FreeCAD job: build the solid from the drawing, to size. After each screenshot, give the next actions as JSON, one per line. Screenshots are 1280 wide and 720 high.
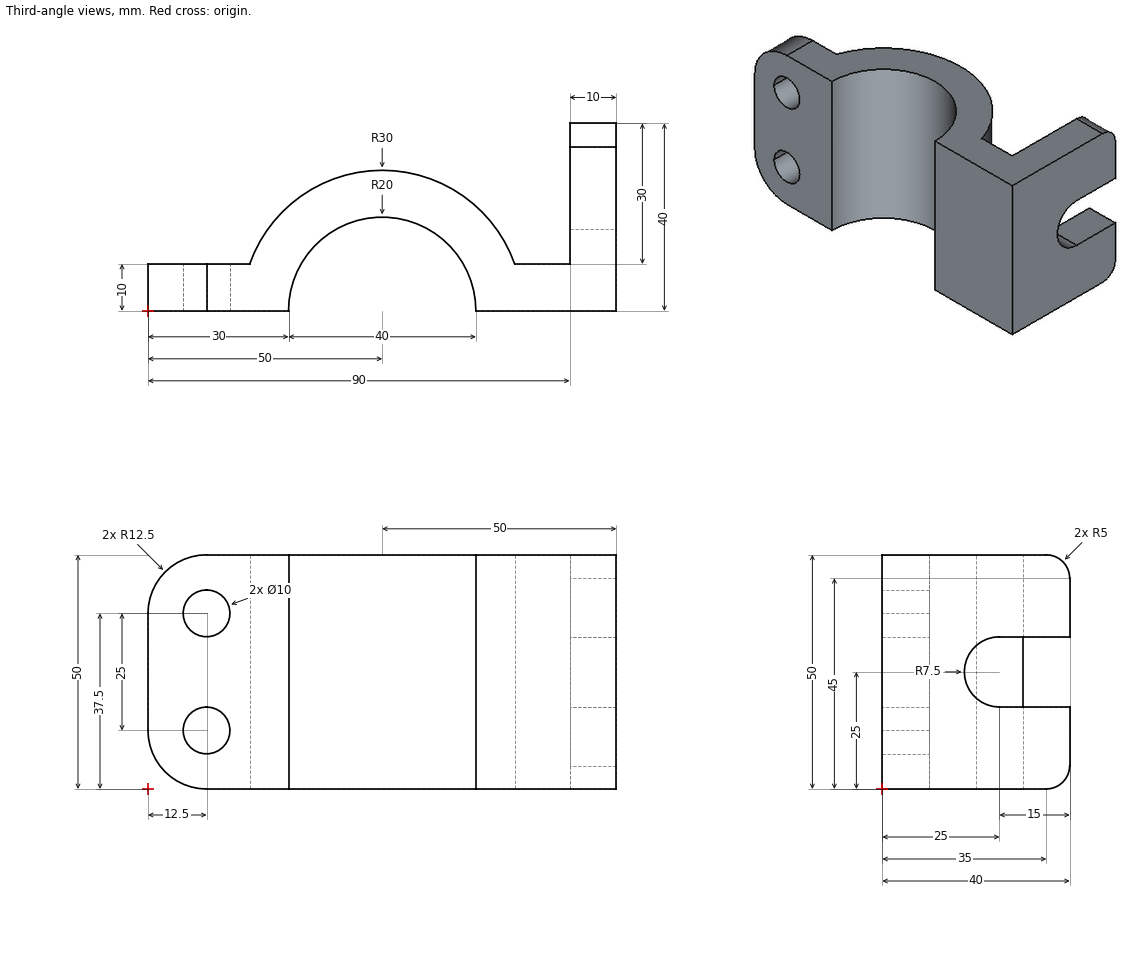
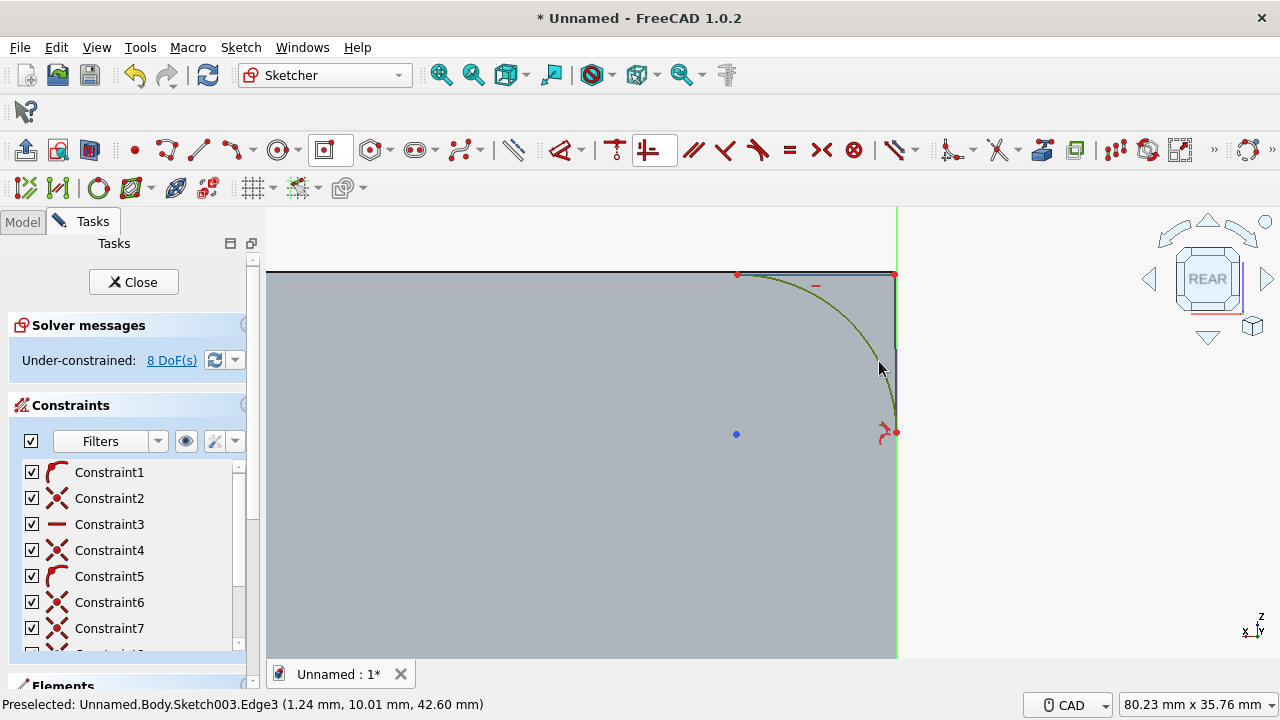
{"action": "left_click", "coordinate": [758, 150]}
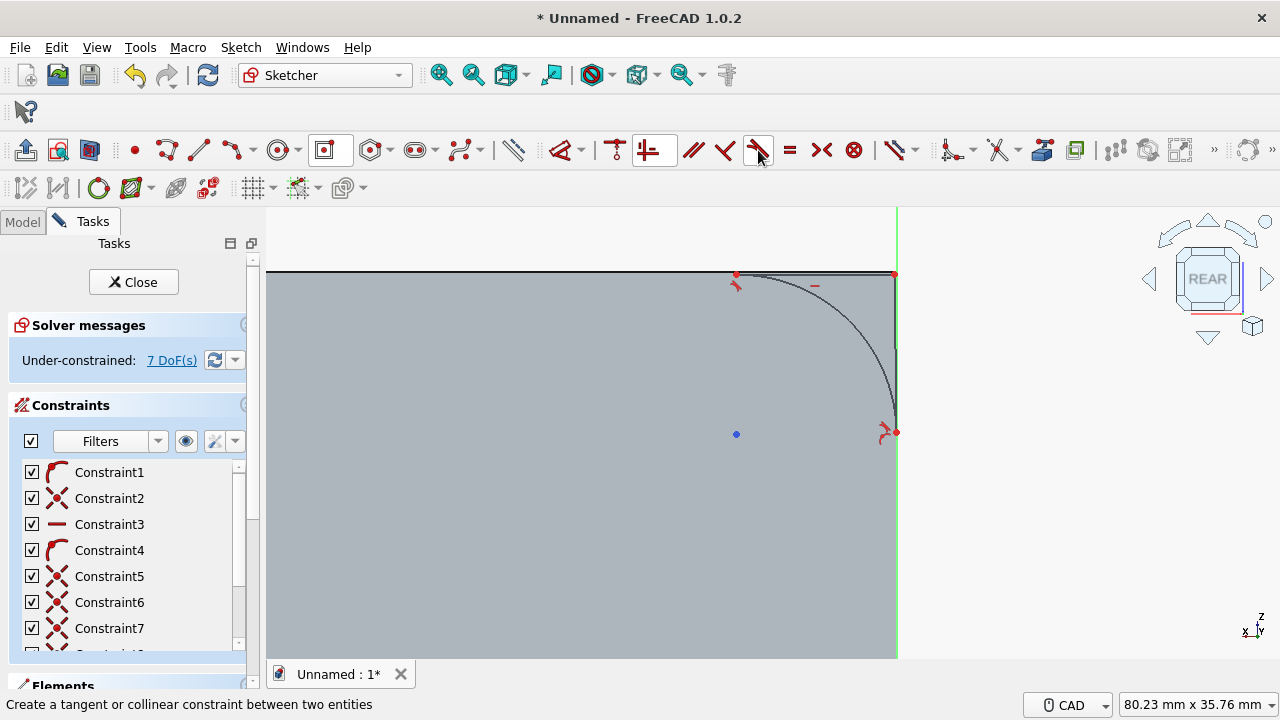
{"action": "scroll", "coordinate": [612, 307], "scroll_direction": "down", "scroll_amount": 4}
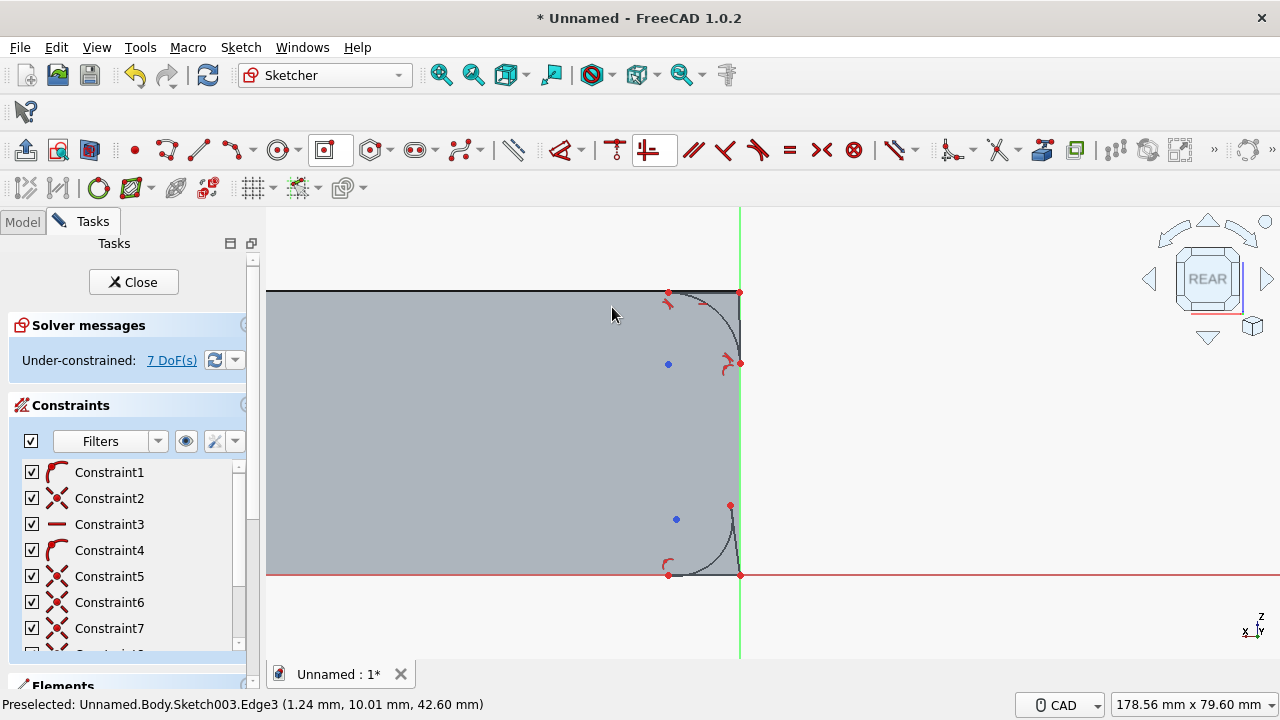
{"action": "left_click", "coordinate": [719, 575]}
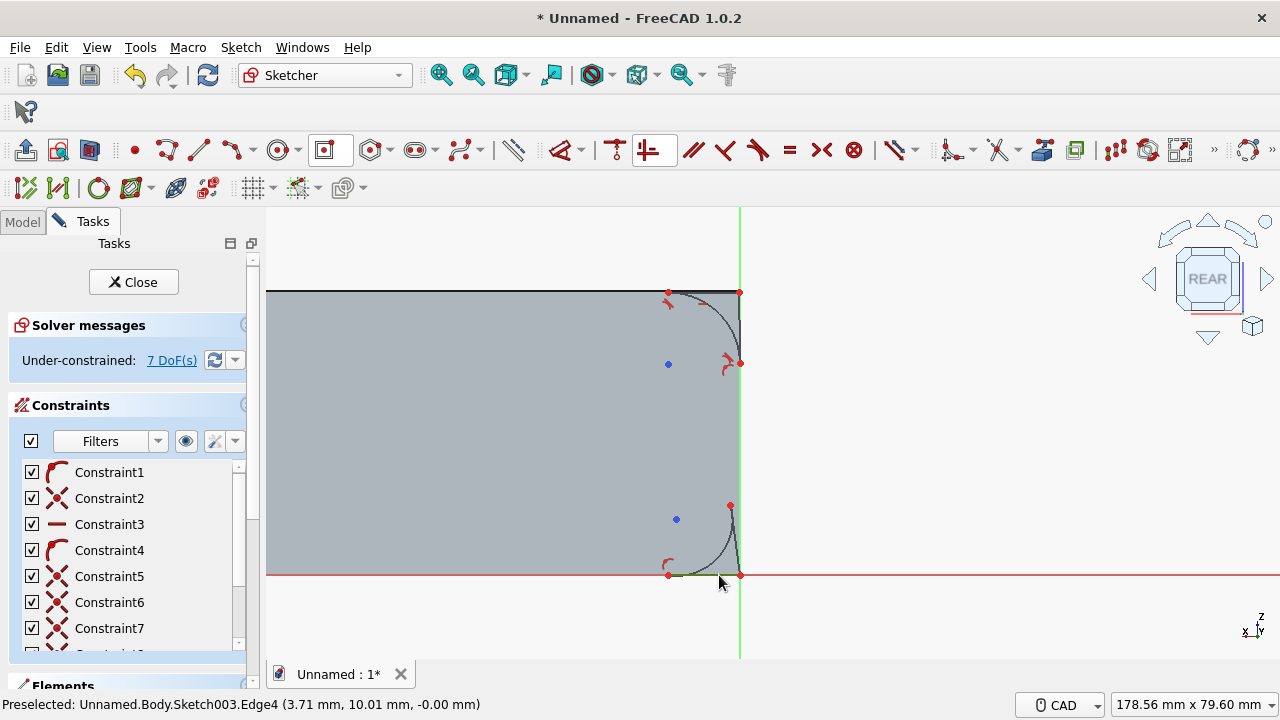
{"action": "left_click", "coordinate": [718, 557]}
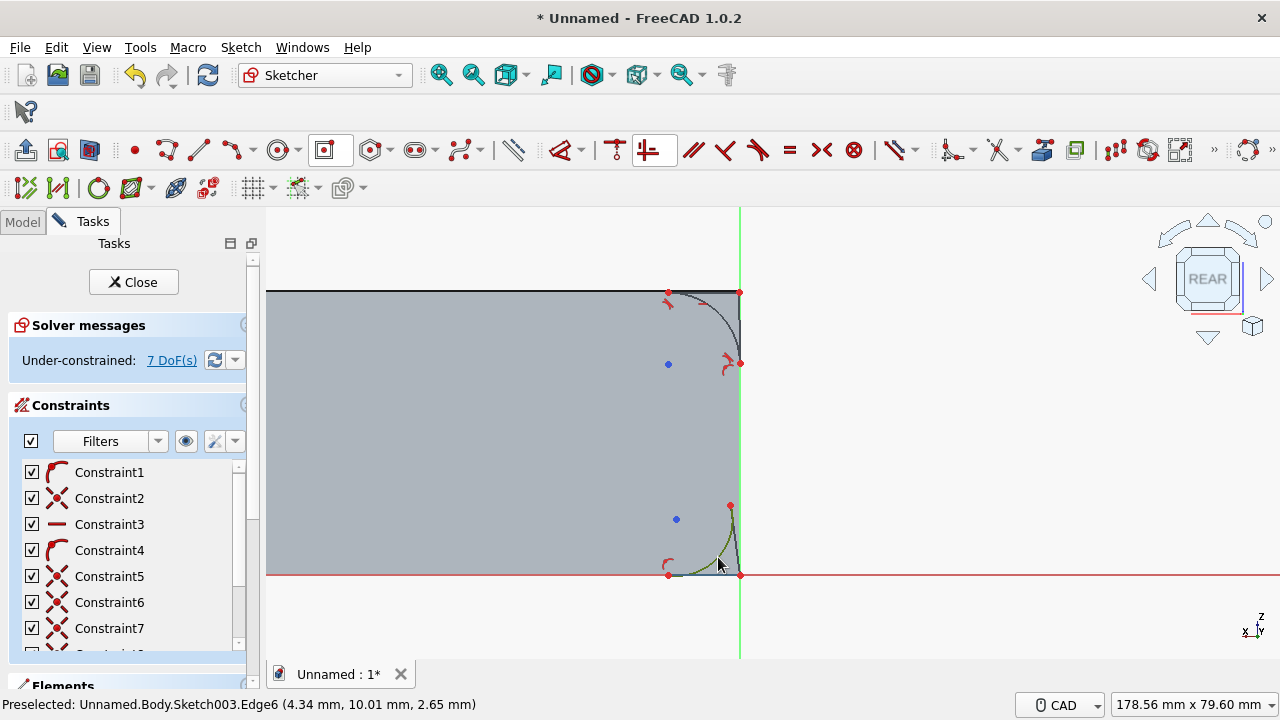
{"action": "left_click", "coordinate": [758, 150]}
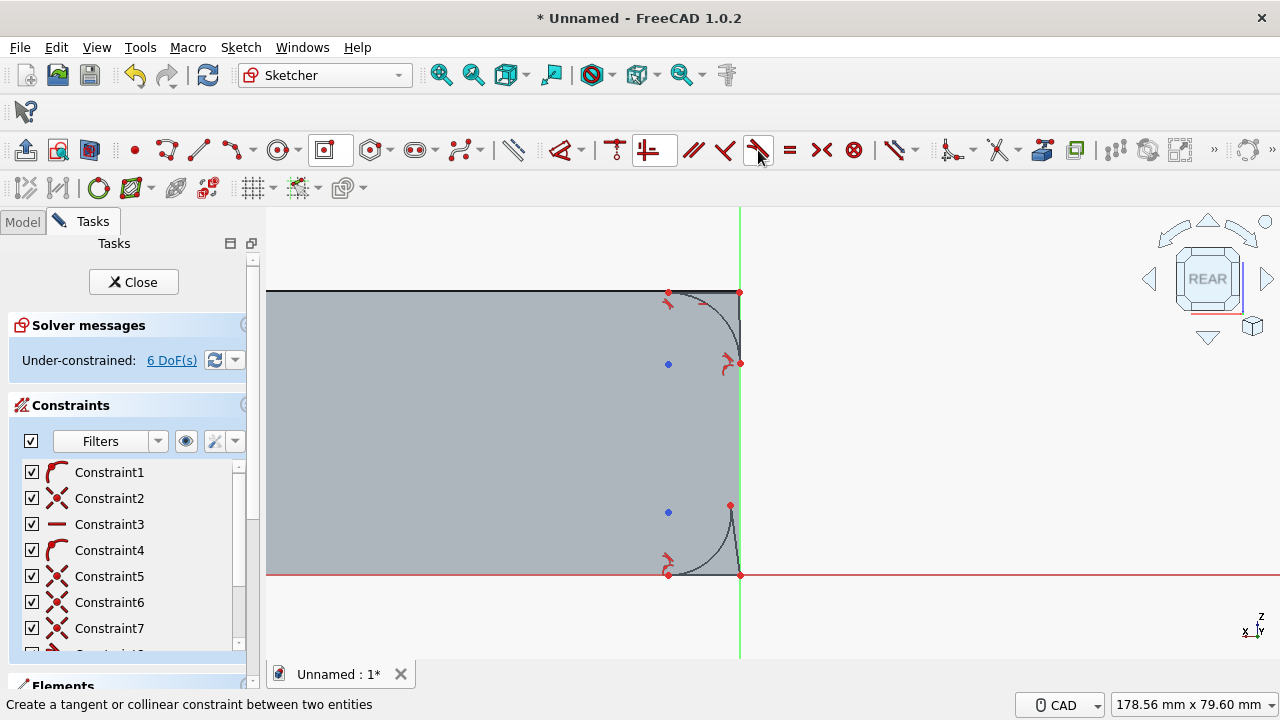
{"action": "left_click", "coordinate": [737, 554]}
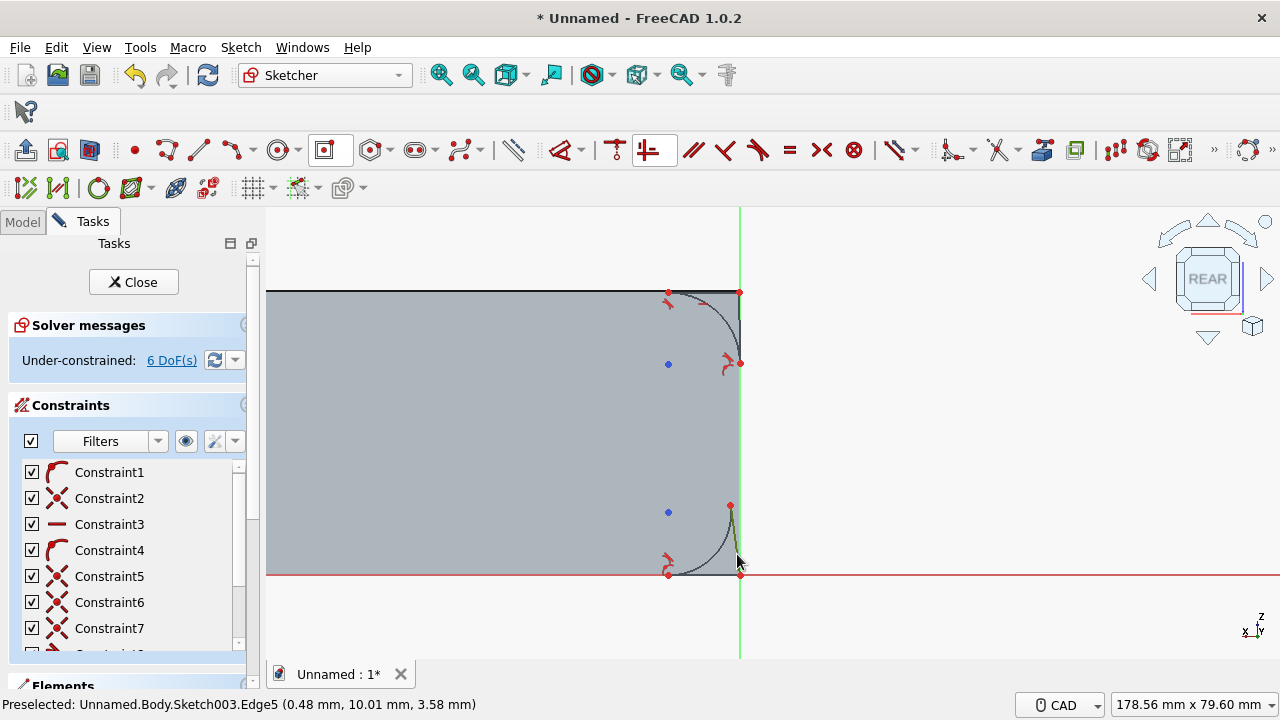
{"action": "left_click", "coordinate": [715, 554]}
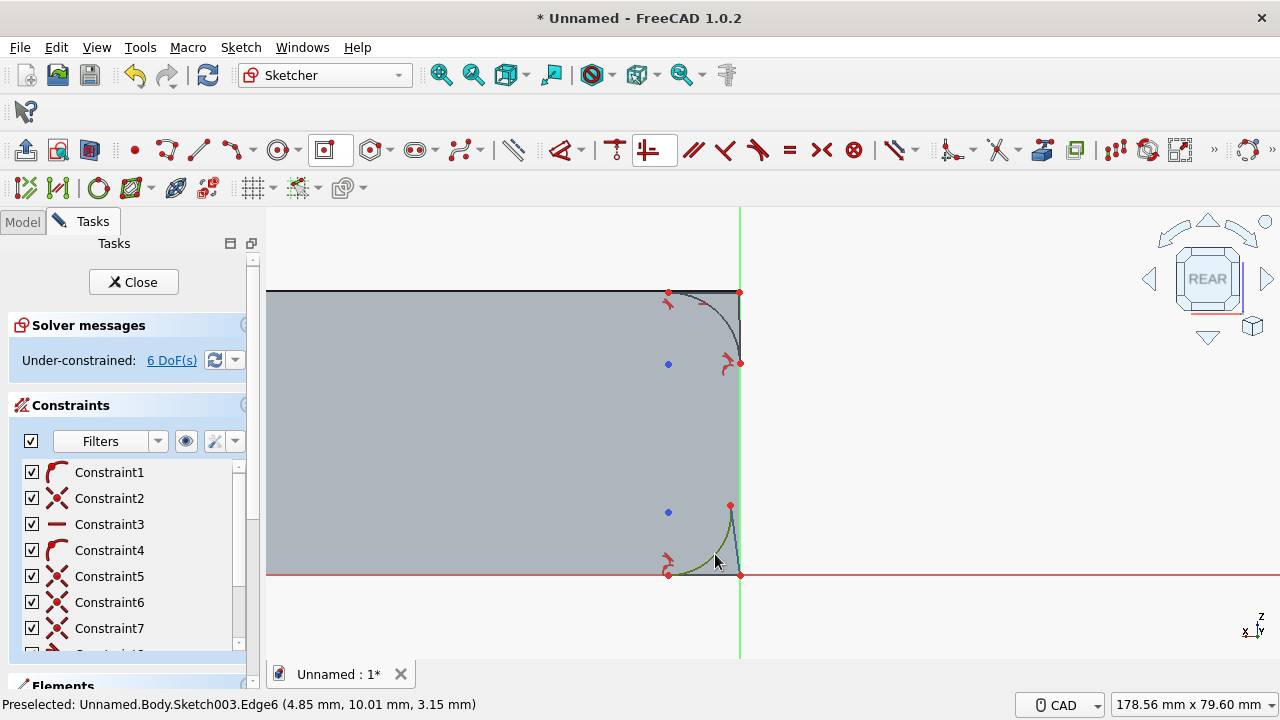
{"action": "left_click", "coordinate": [758, 150]}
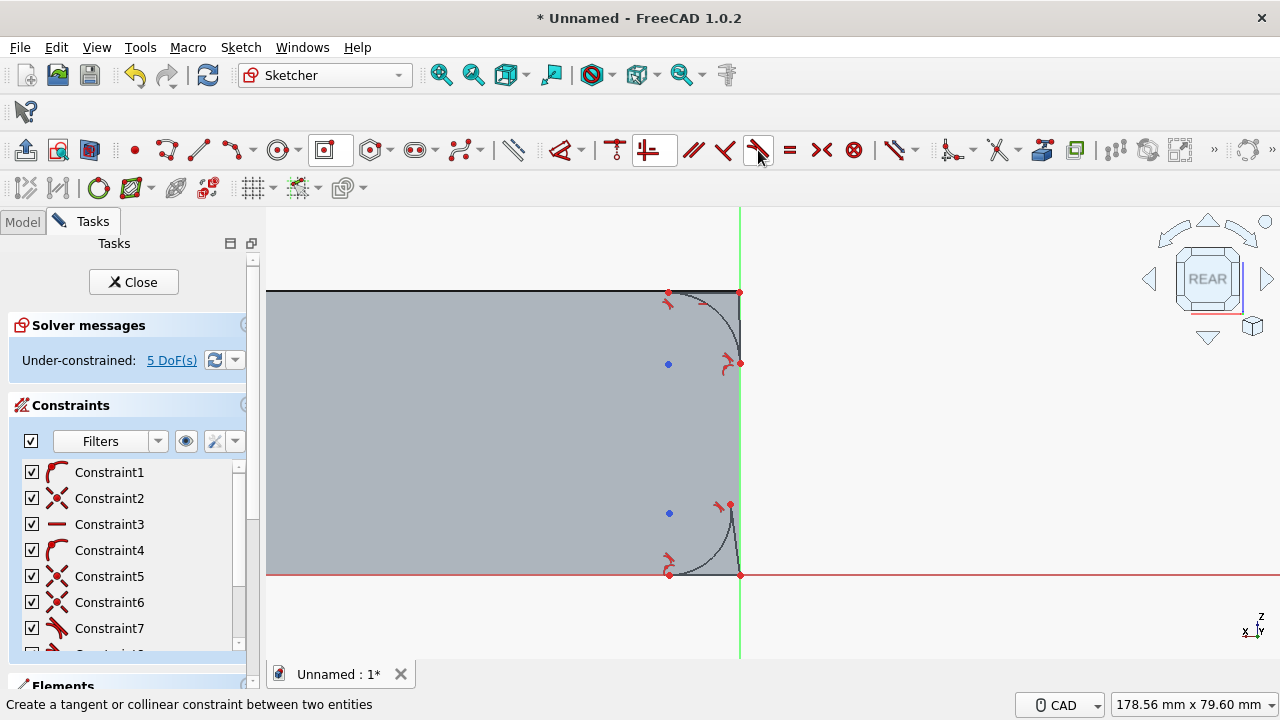
{"action": "left_click", "coordinate": [739, 314]}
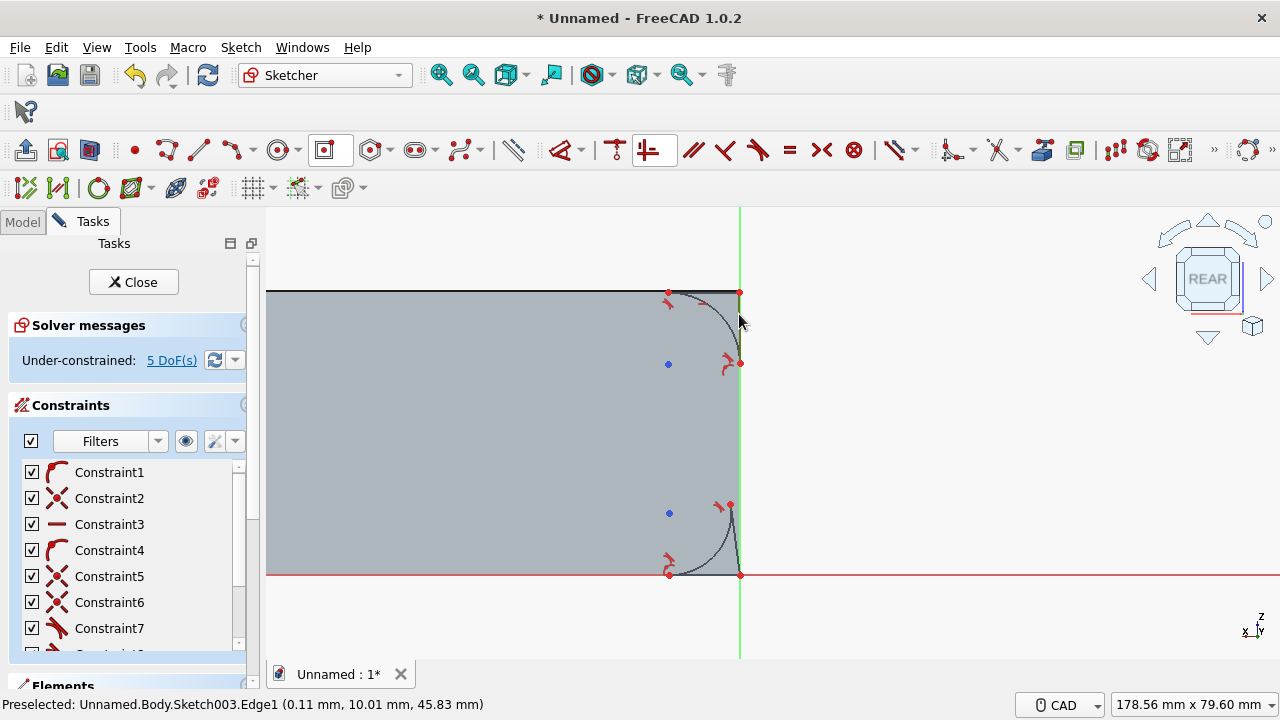
{"action": "left_click", "coordinate": [672, 150]}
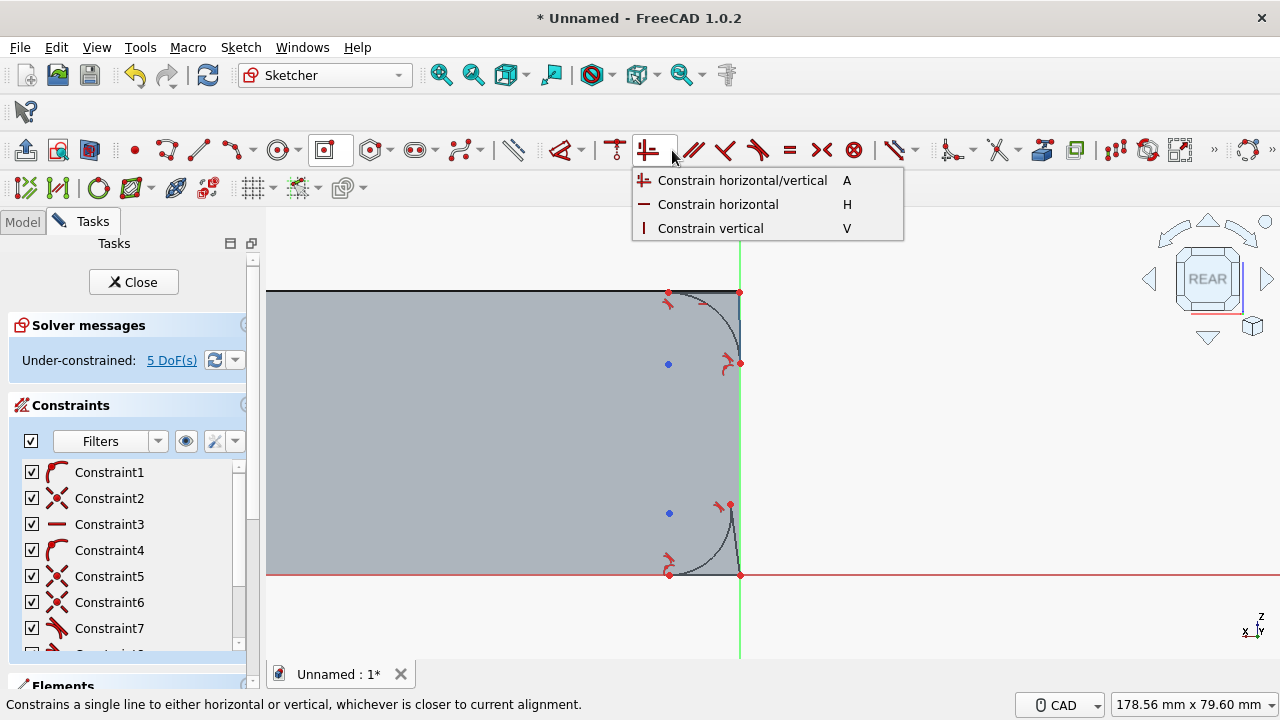
{"action": "left_click", "coordinate": [768, 228]}